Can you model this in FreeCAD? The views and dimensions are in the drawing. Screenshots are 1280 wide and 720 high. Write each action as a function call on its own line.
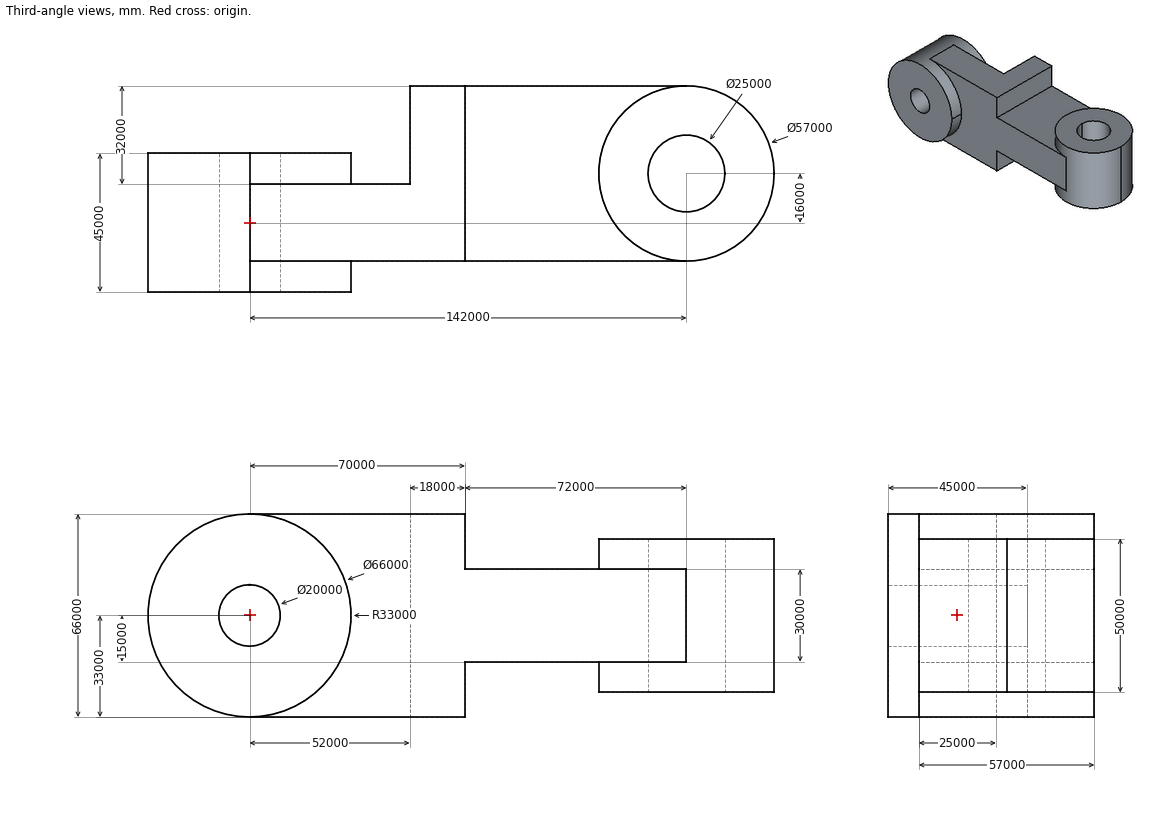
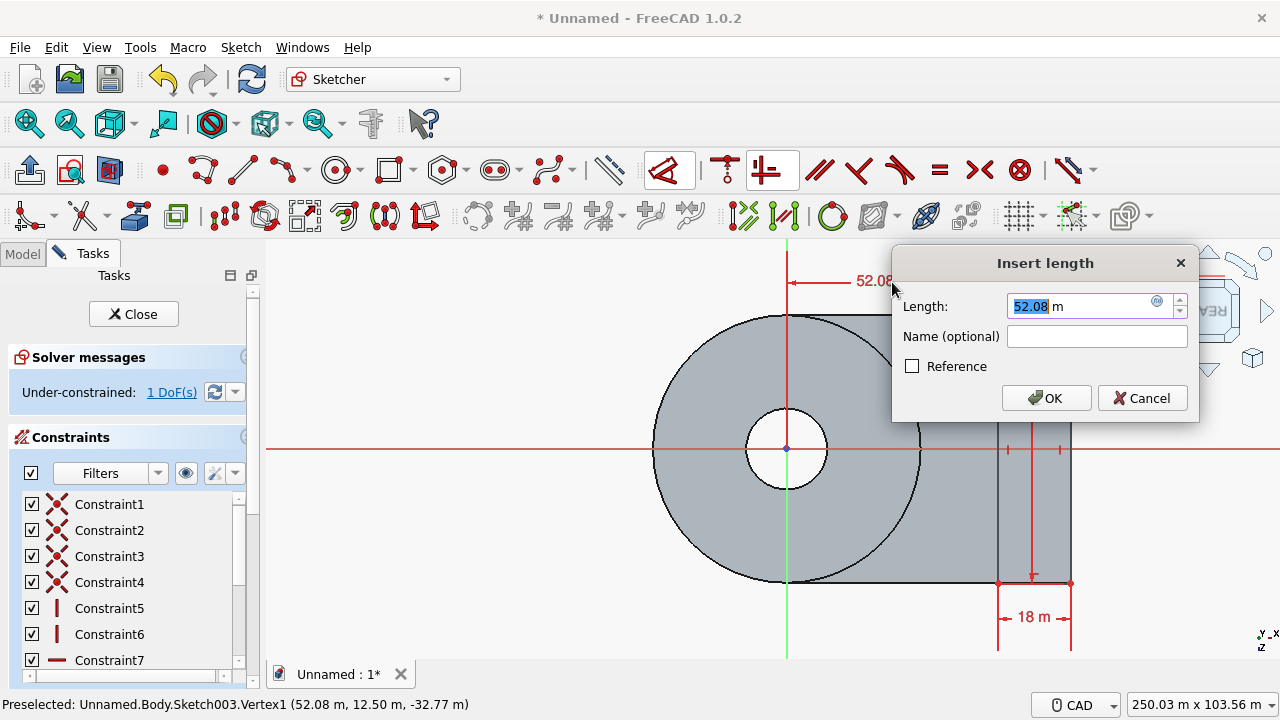
key(ctrl+a)
text(52000 mm)
key(Return)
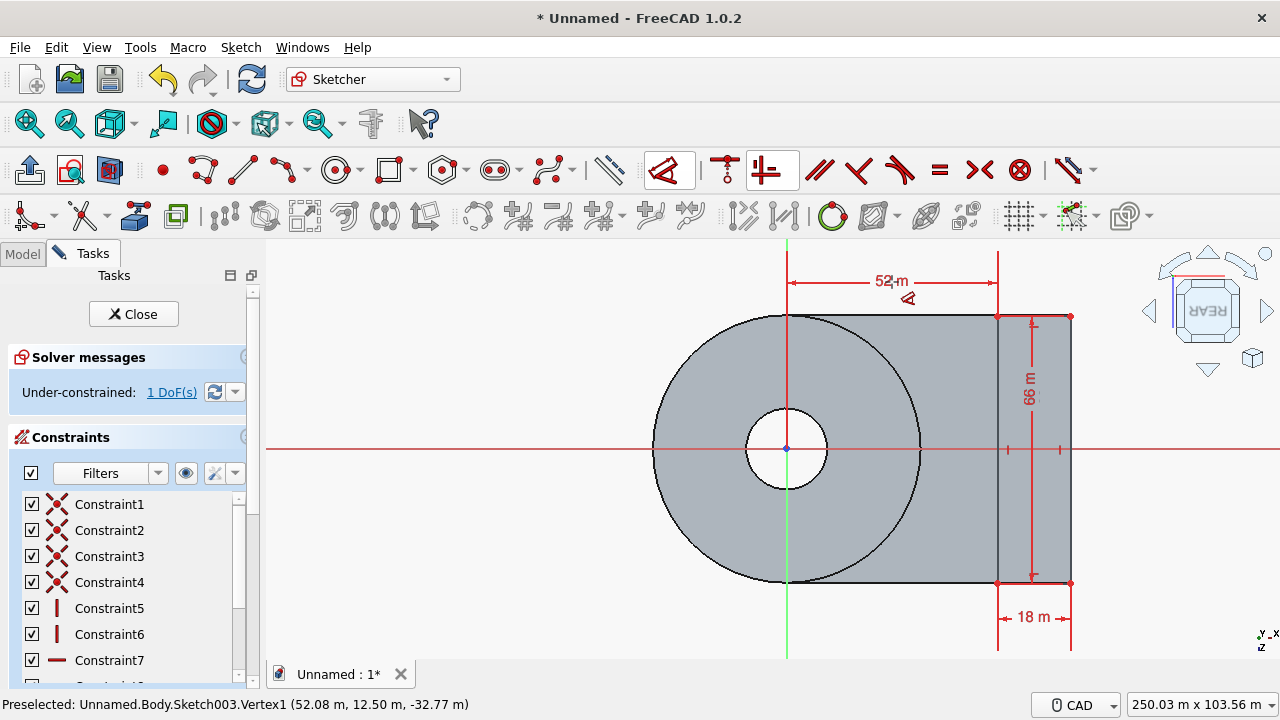
click(998, 316)
click(753, 383)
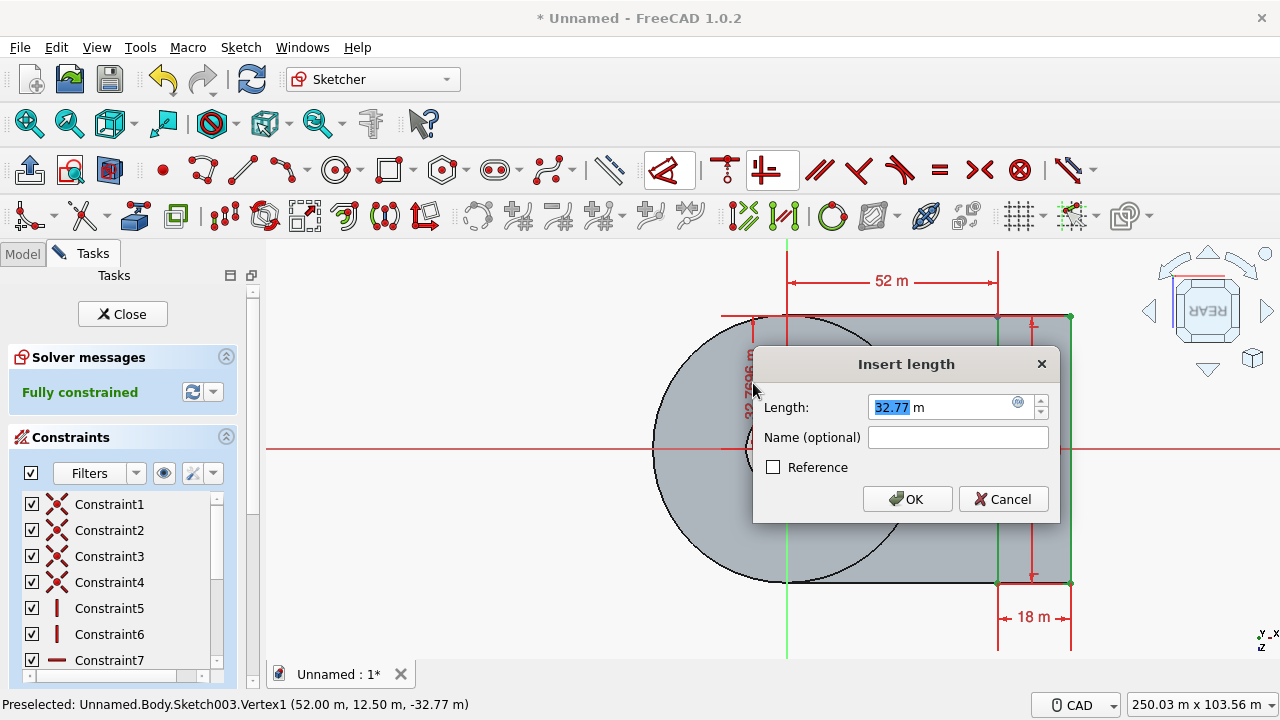
key(ctrl+a)
text(33000 mm)
key(Return)
key(Escape)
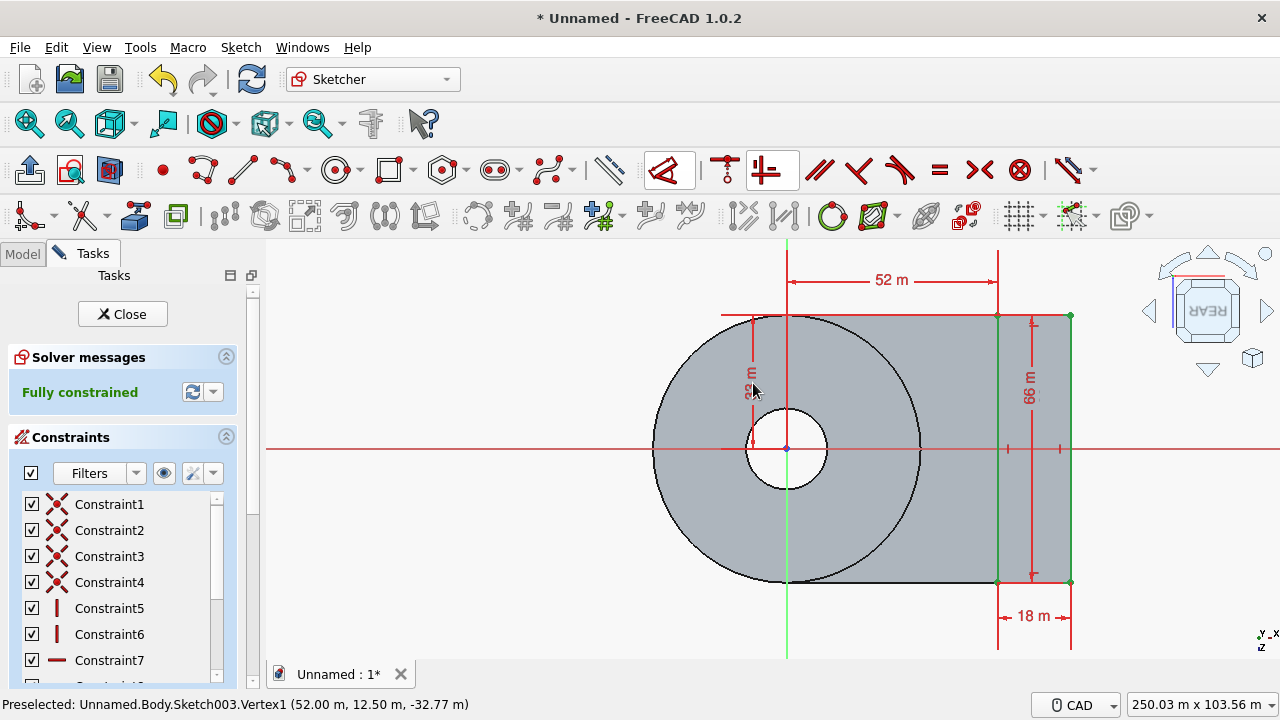
click(123, 314)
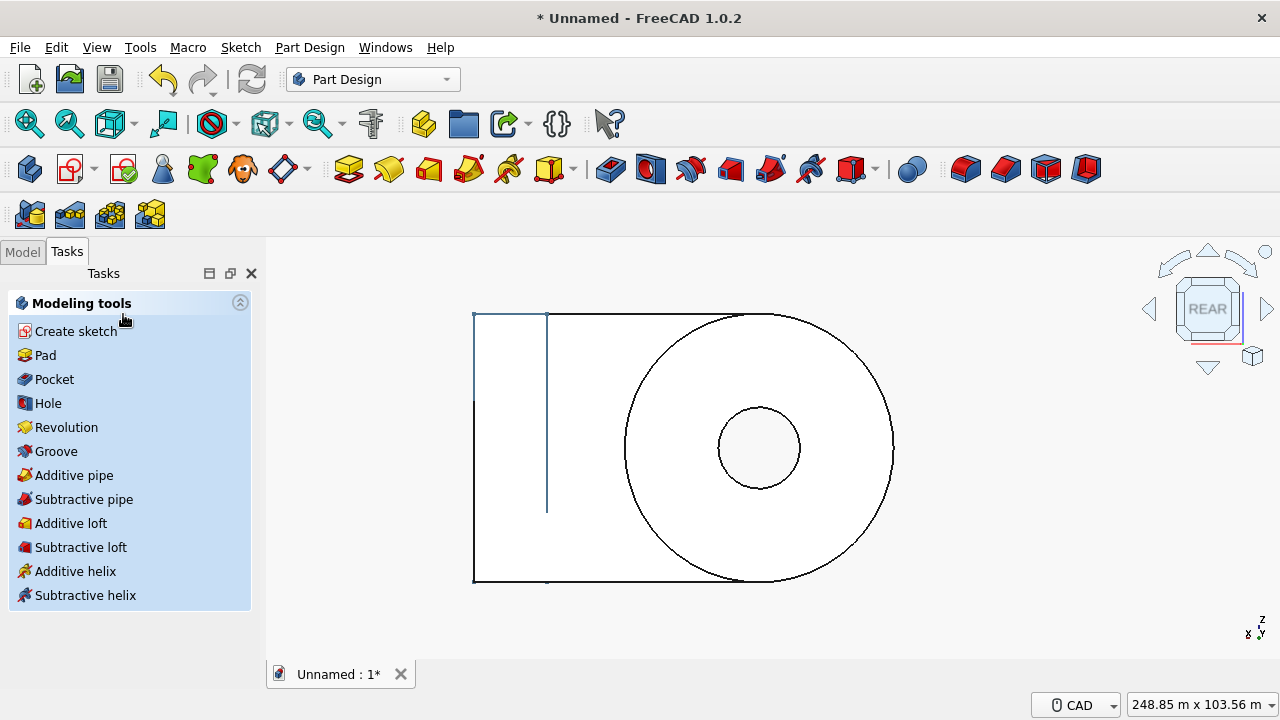
click(350, 170)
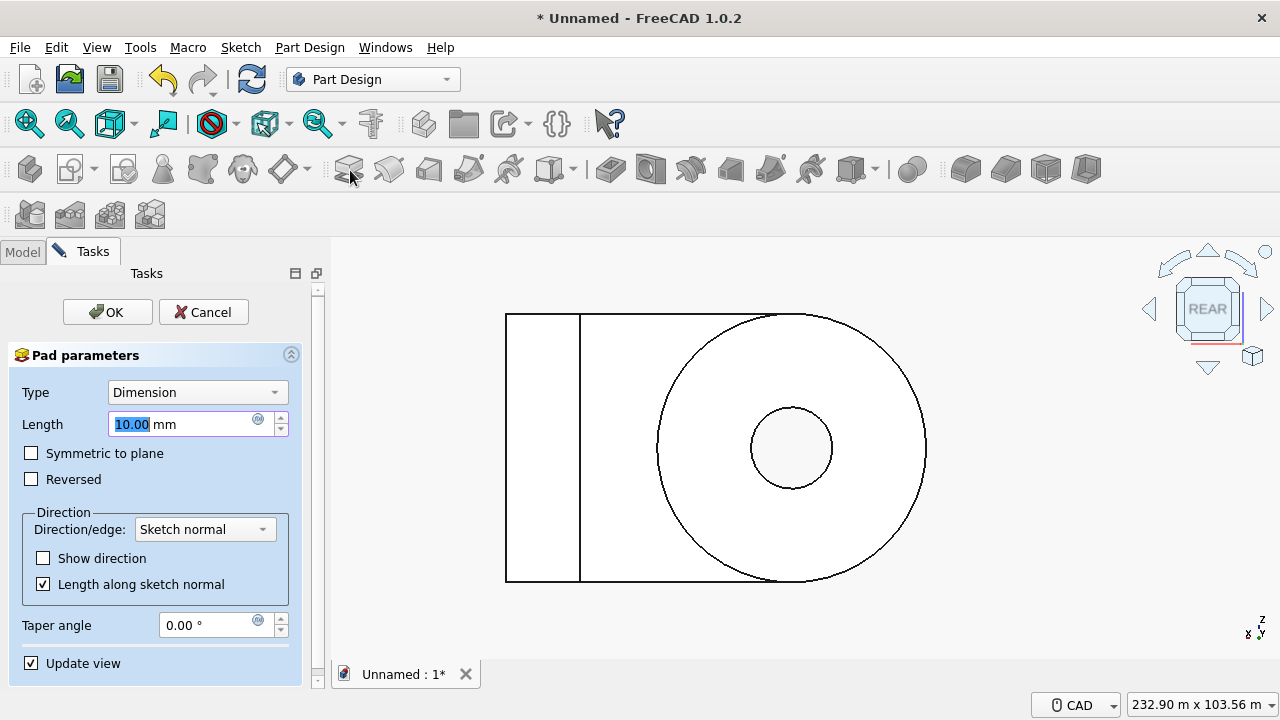
text(32000)
key(Tab)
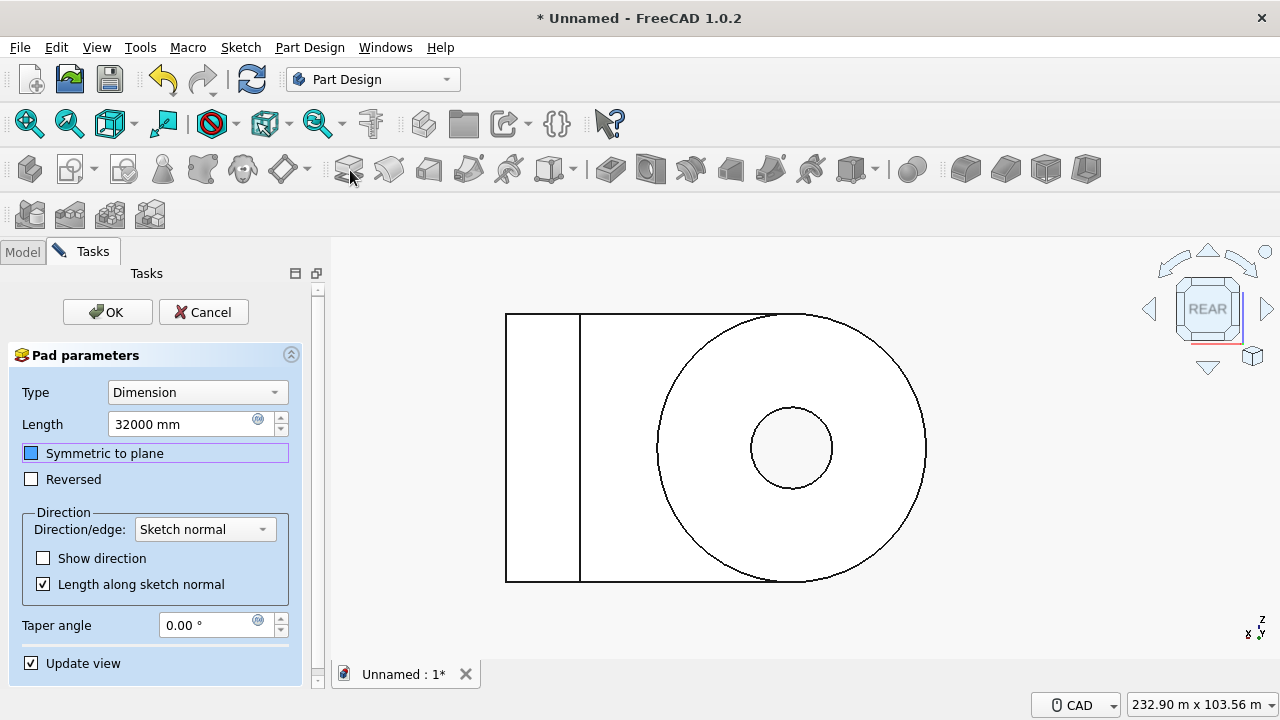
click(108, 312)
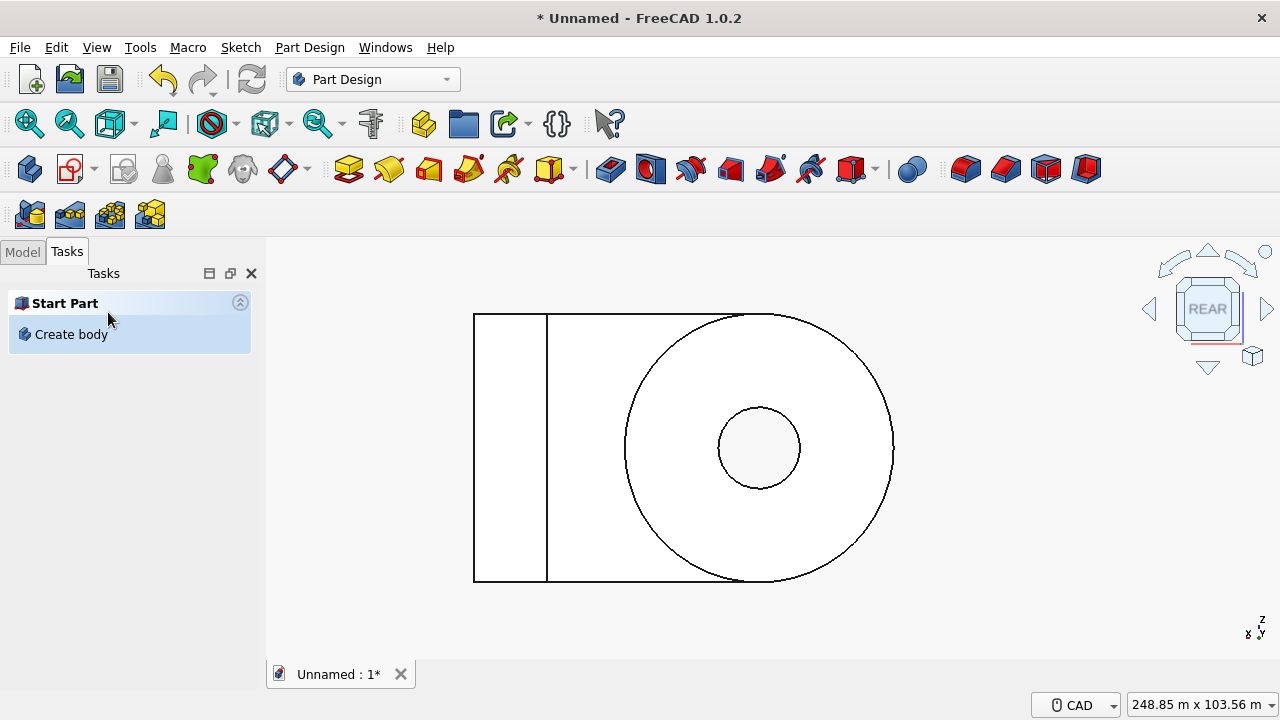
click(511, 370)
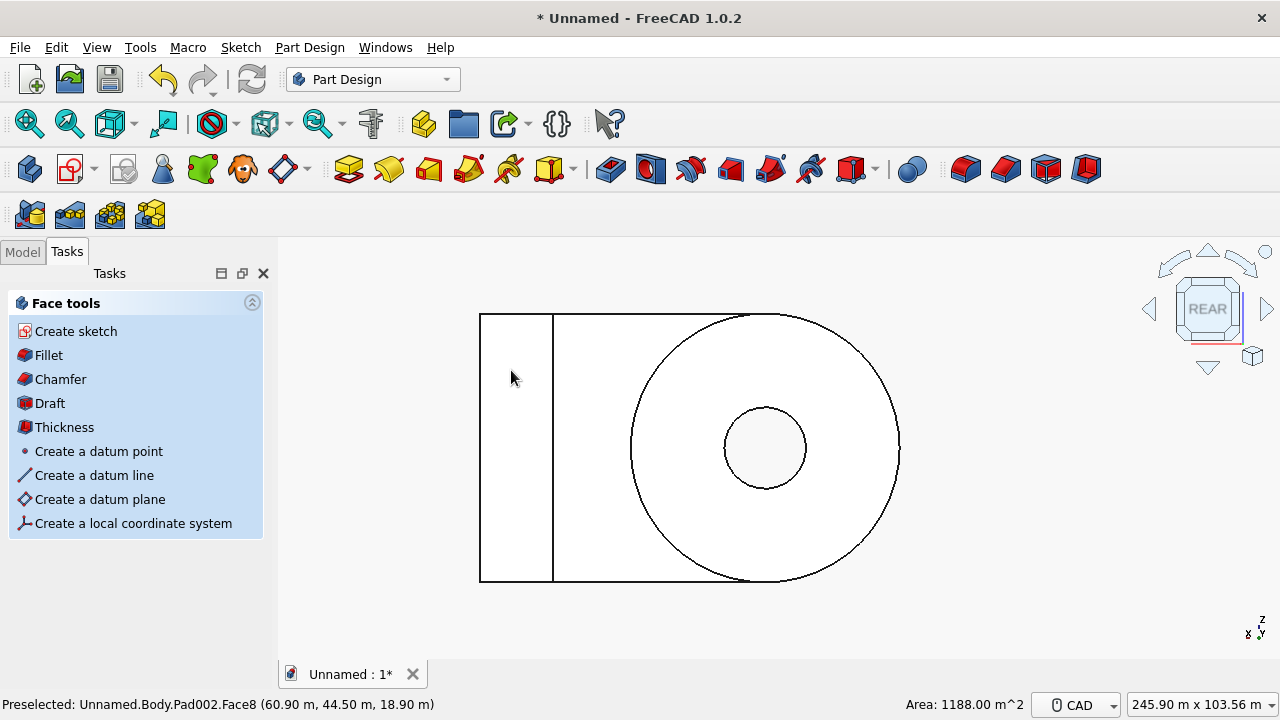
click(70, 170)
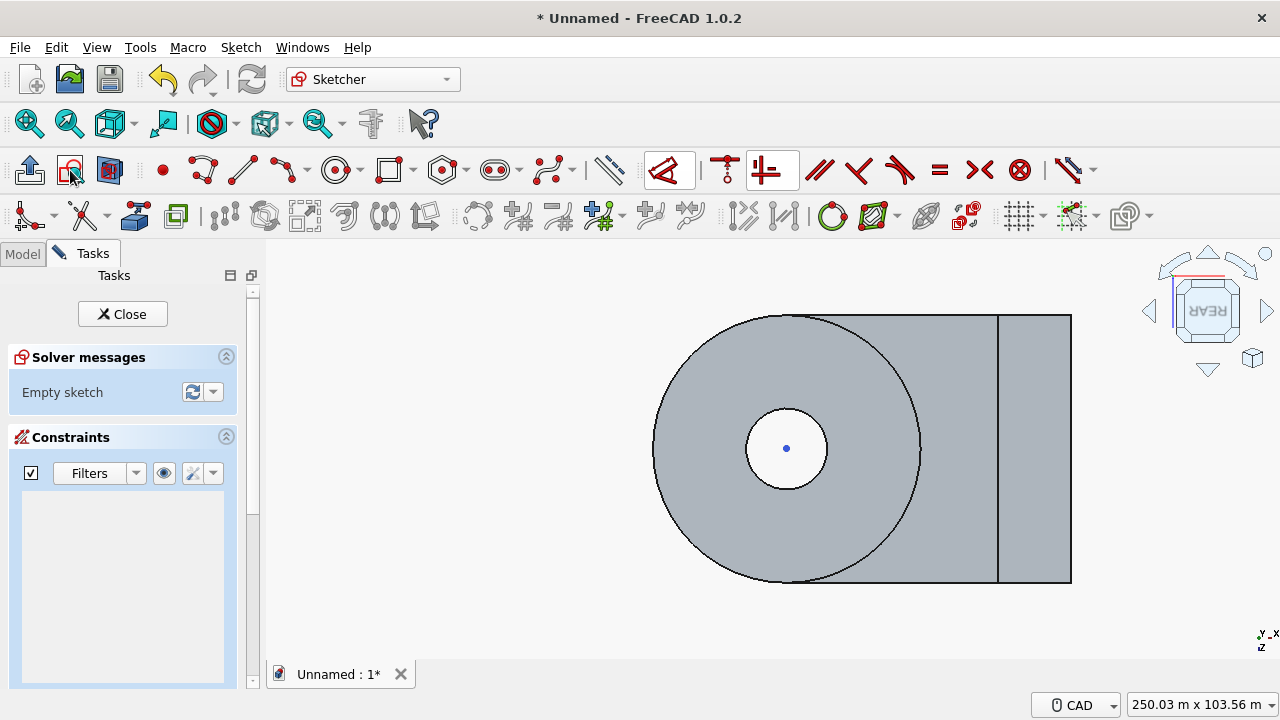
scroll(294, 449, down, 2)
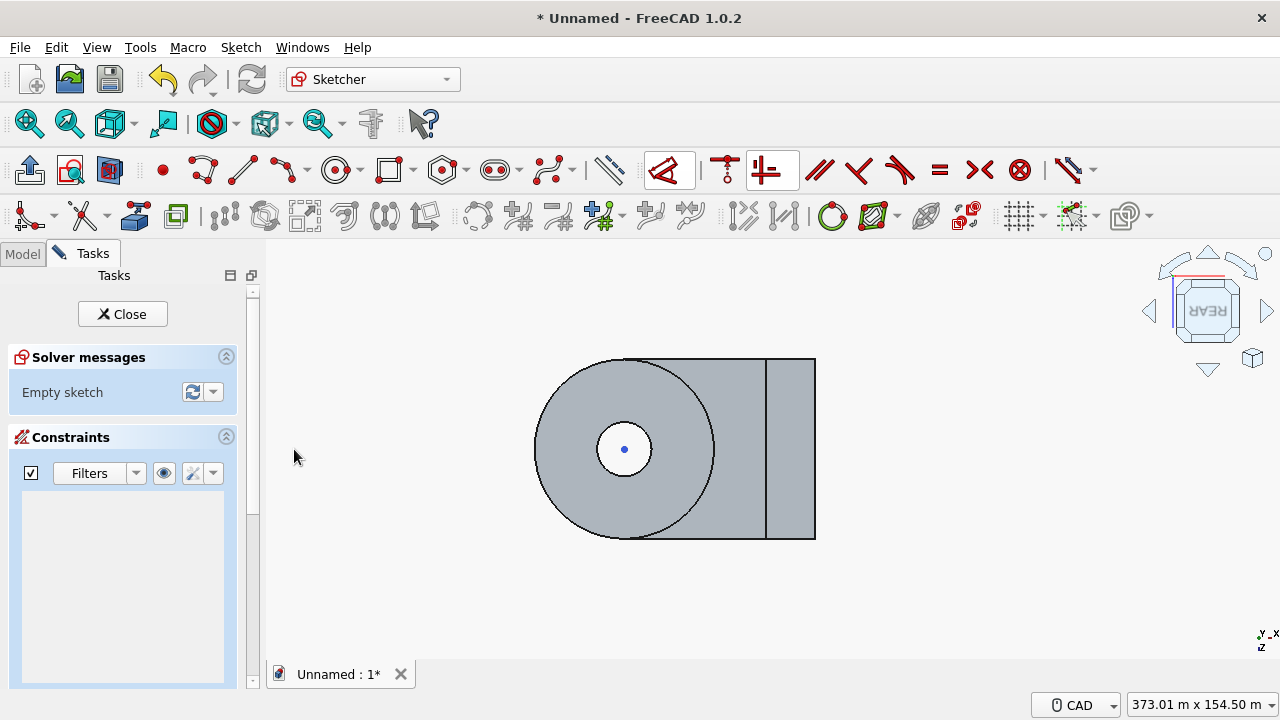
scroll(1047, 450, up, 2)